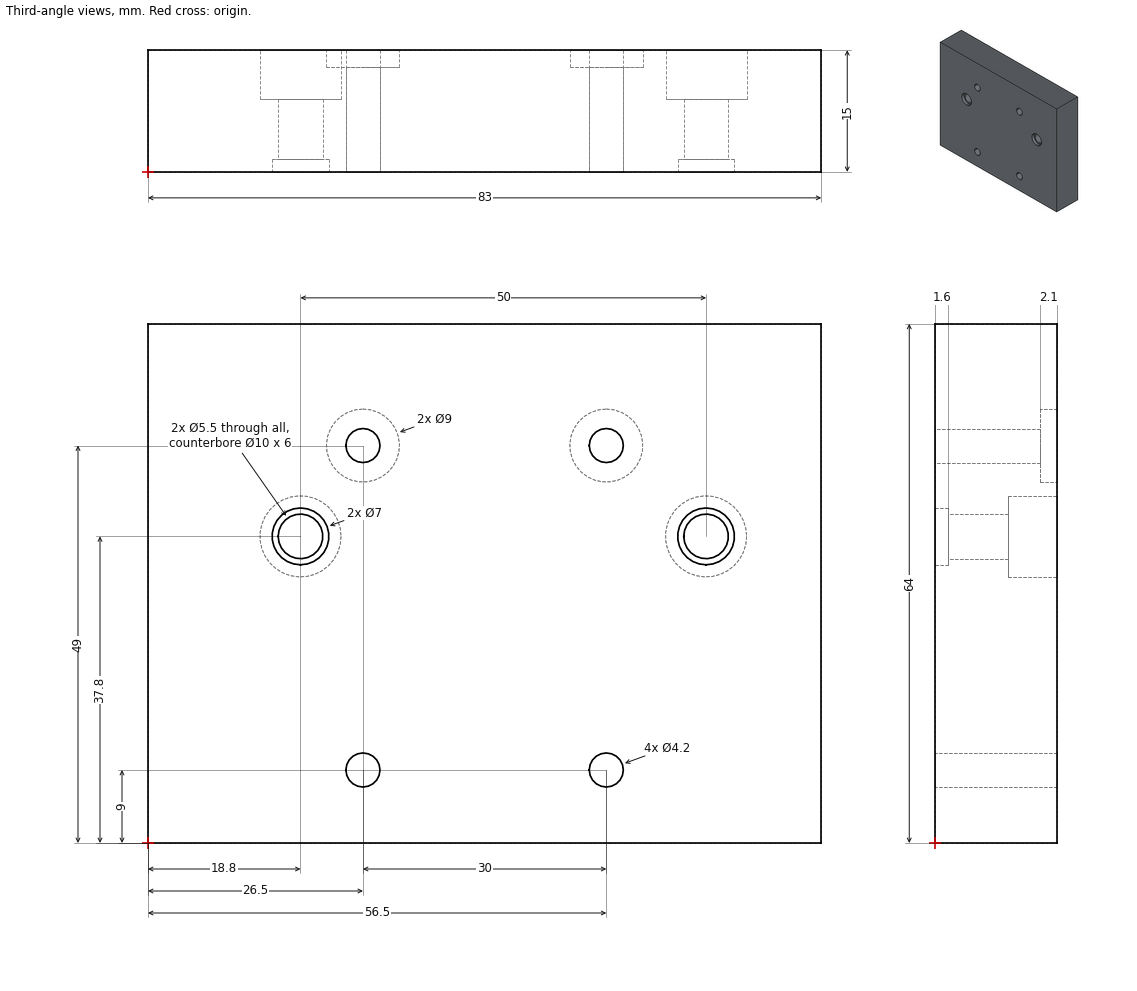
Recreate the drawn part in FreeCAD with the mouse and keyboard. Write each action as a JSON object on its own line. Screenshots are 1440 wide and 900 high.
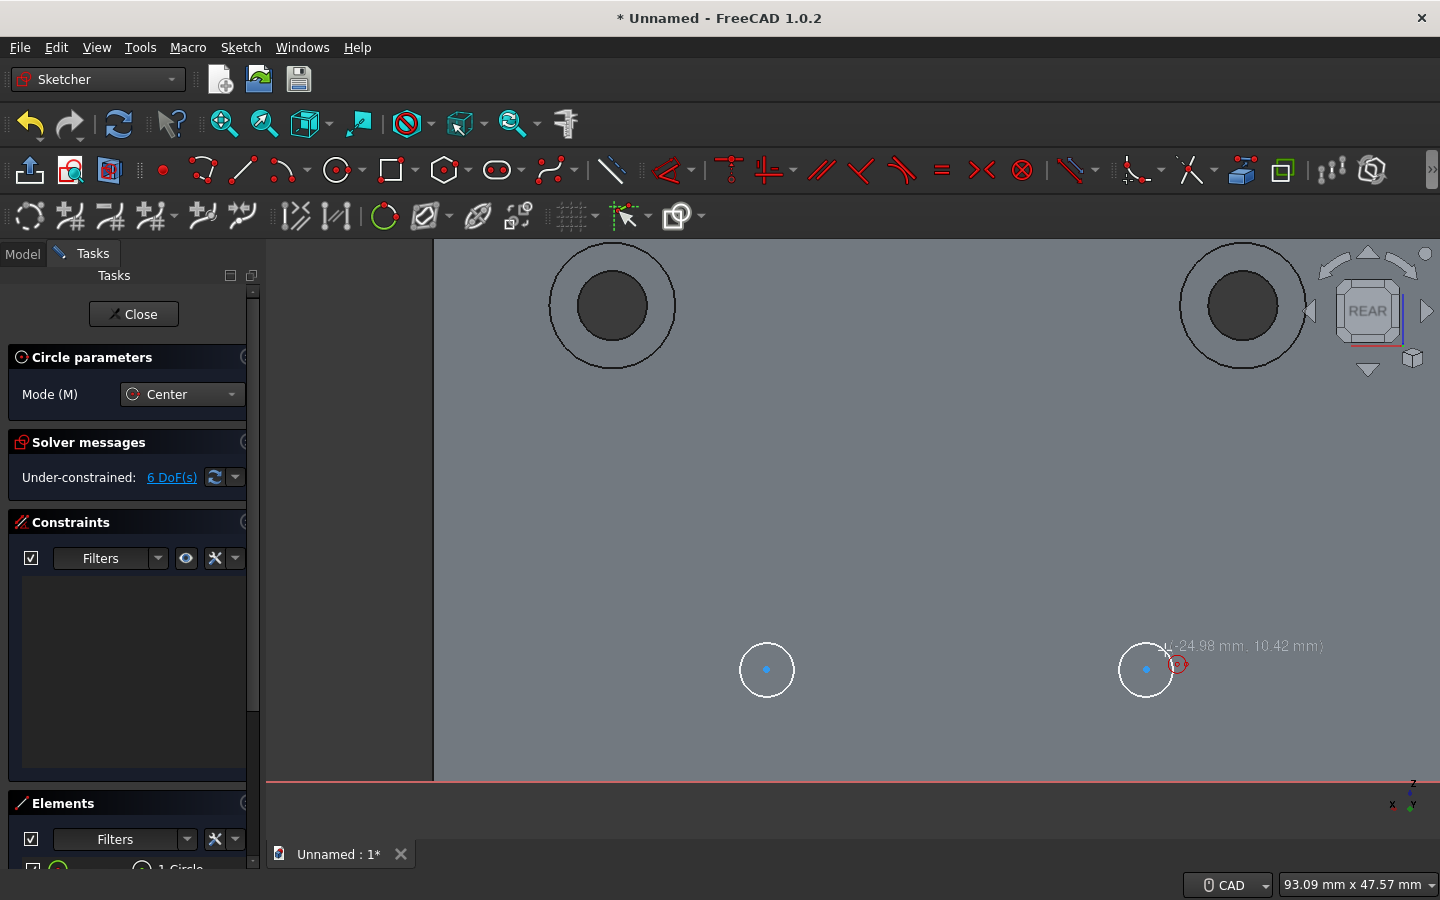
{"action": "scroll", "coordinate": [388, 635], "scroll_direction": "down", "scroll_amount": 3}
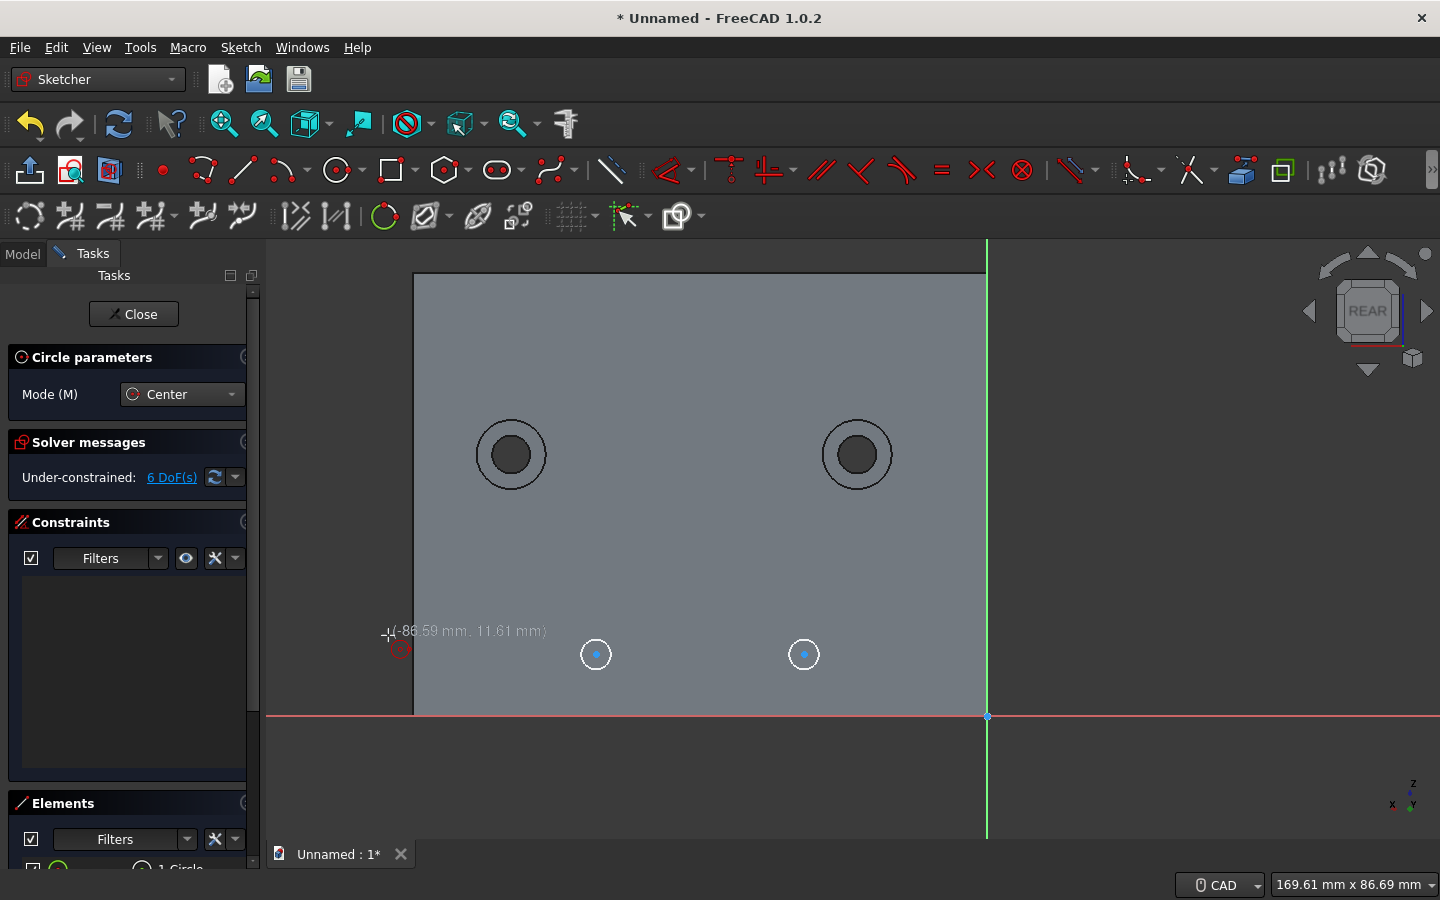
{"action": "scroll", "coordinate": [804, 377], "scroll_direction": "up", "scroll_amount": 3}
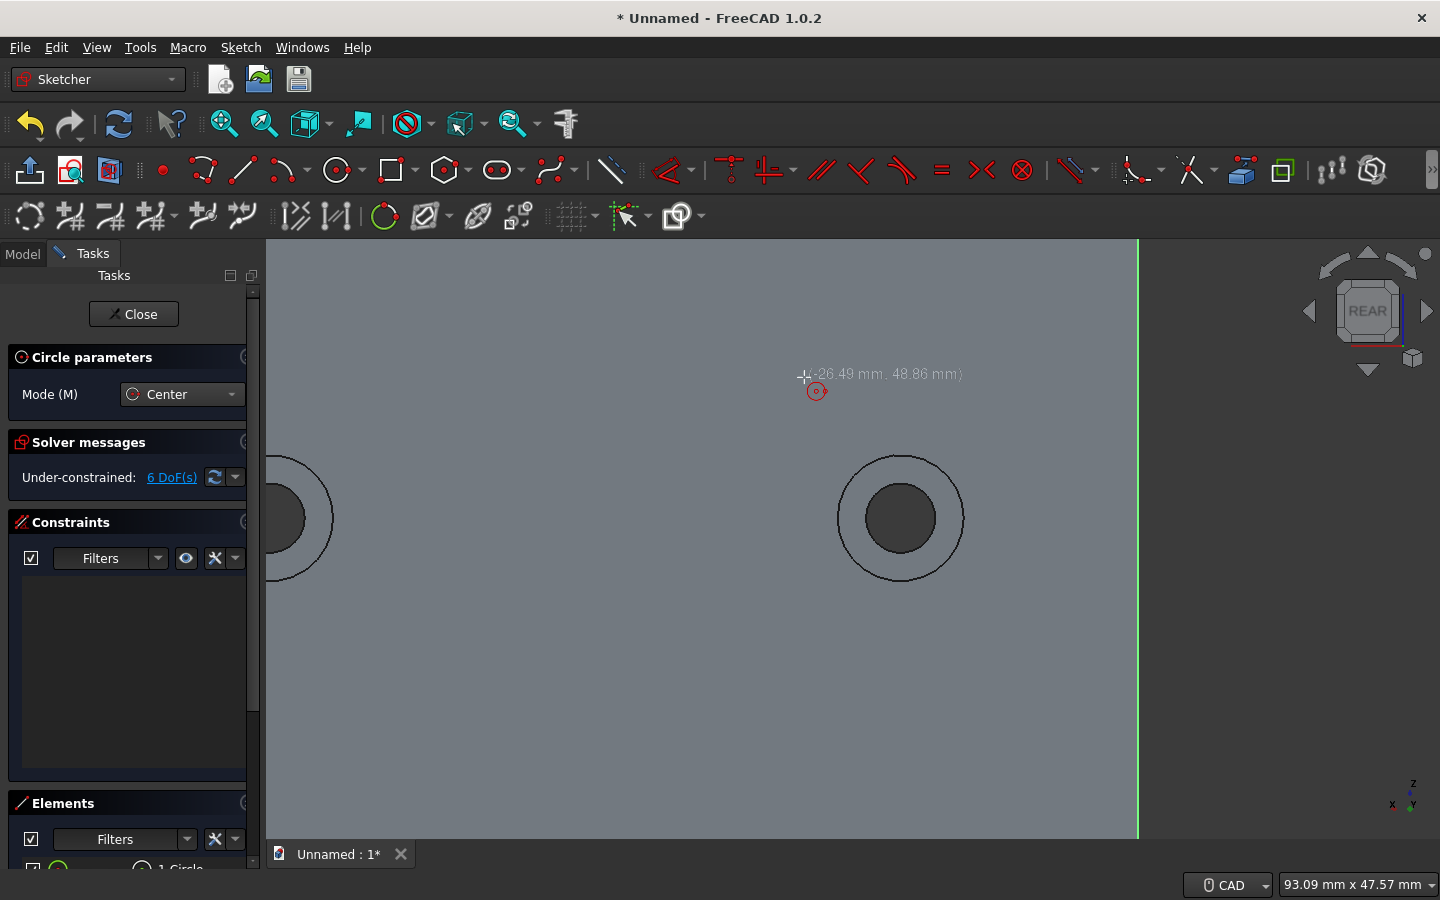
{"action": "left_click", "coordinate": [804, 377]}
{"action": "left_click", "coordinate": [822, 358]}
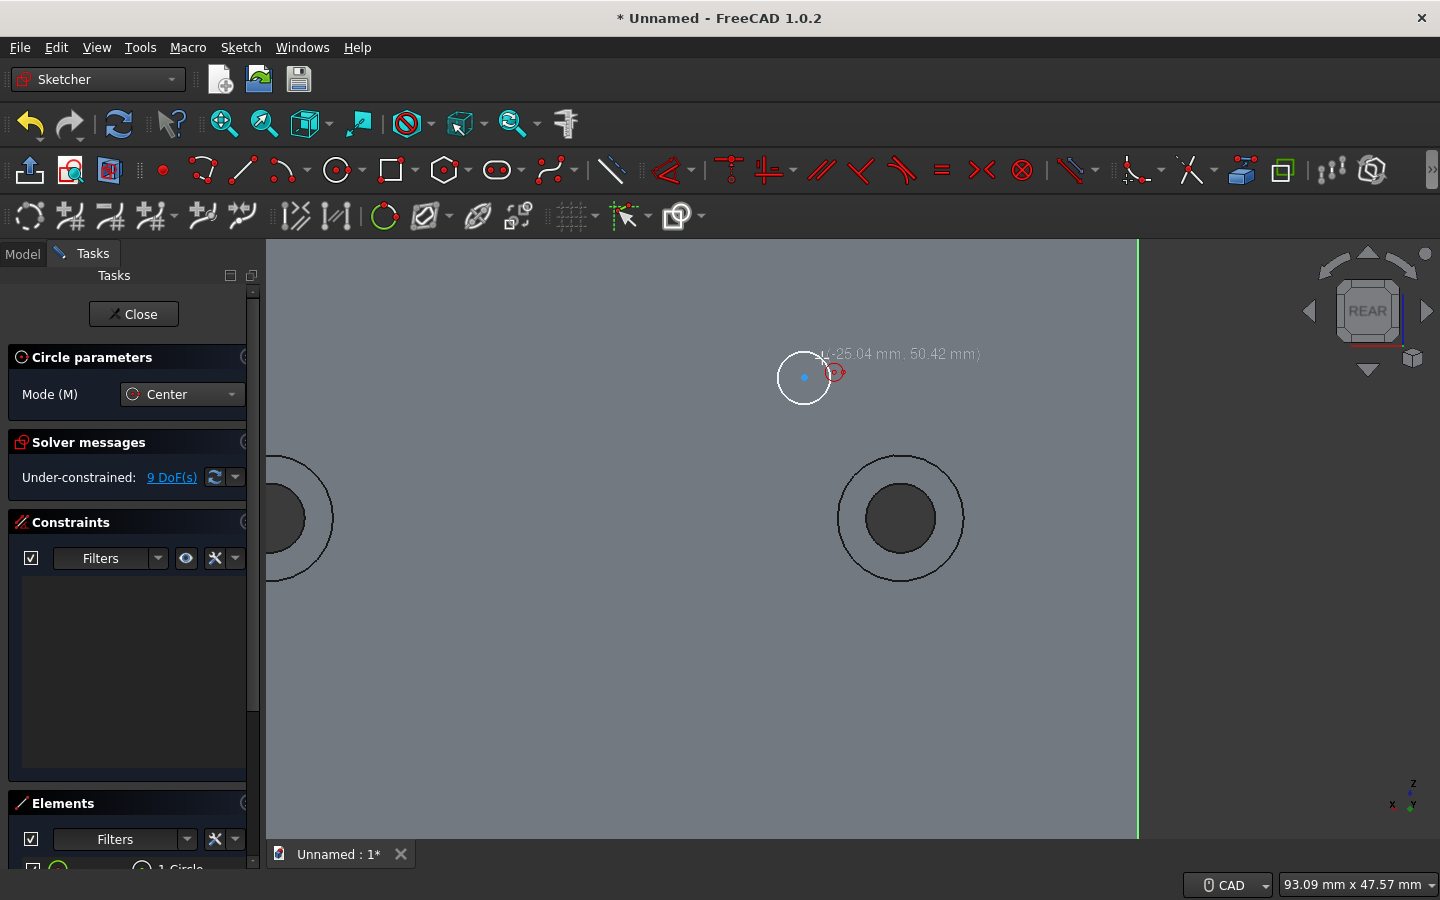
{"action": "left_click", "coordinate": [425, 377]}
{"action": "left_click", "coordinate": [444, 358]}
{"action": "key", "text": "Escape"}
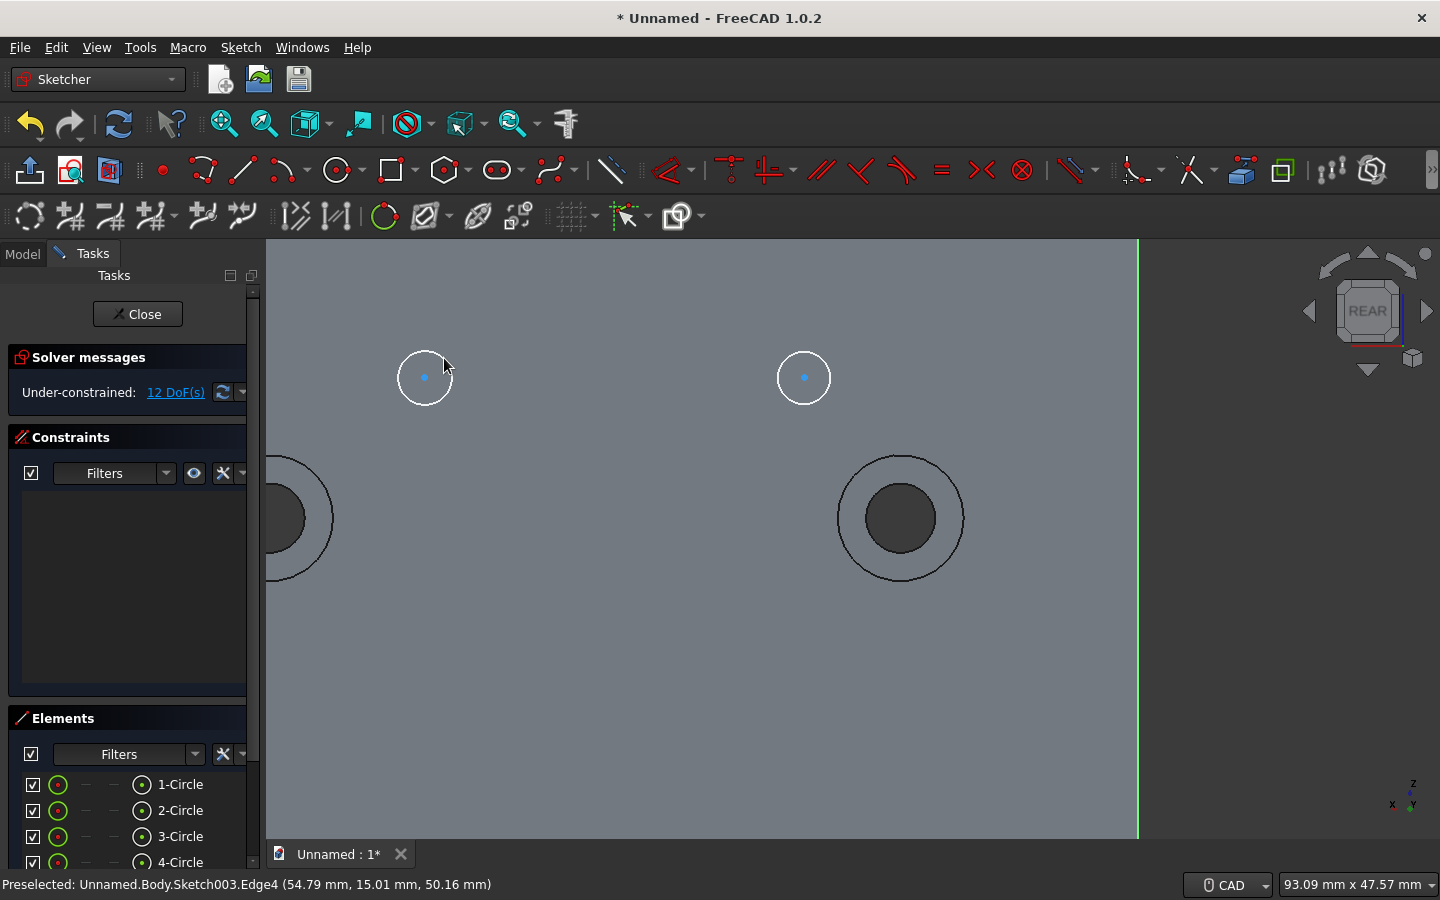
{"action": "scroll", "coordinate": [804, 376], "scroll_direction": "down", "scroll_amount": 3}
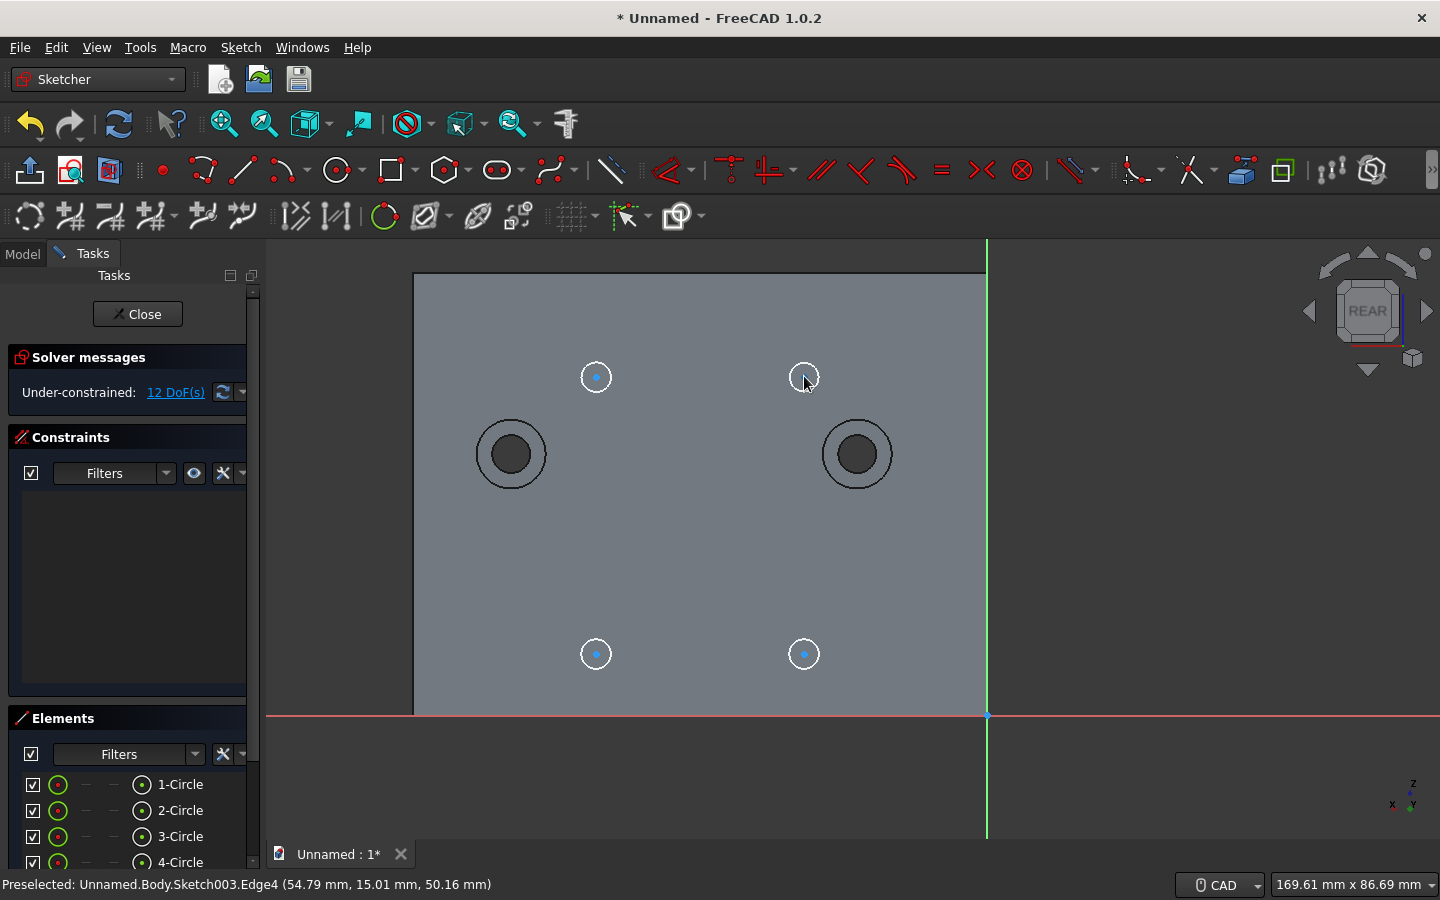
{"action": "left_click", "coordinate": [606, 644]}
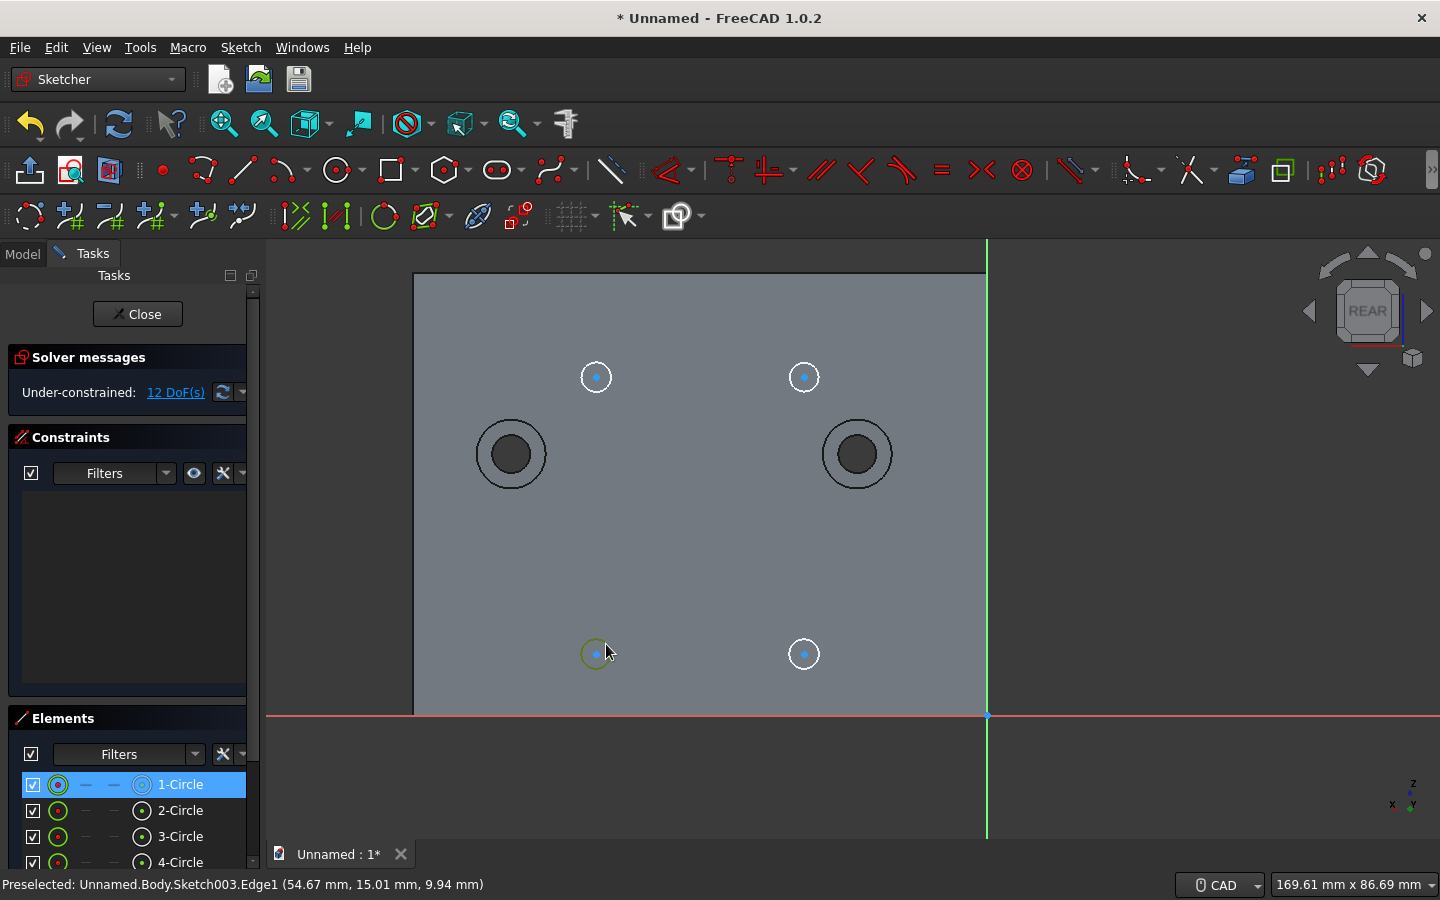
{"action": "left_click", "coordinate": [814, 644]}